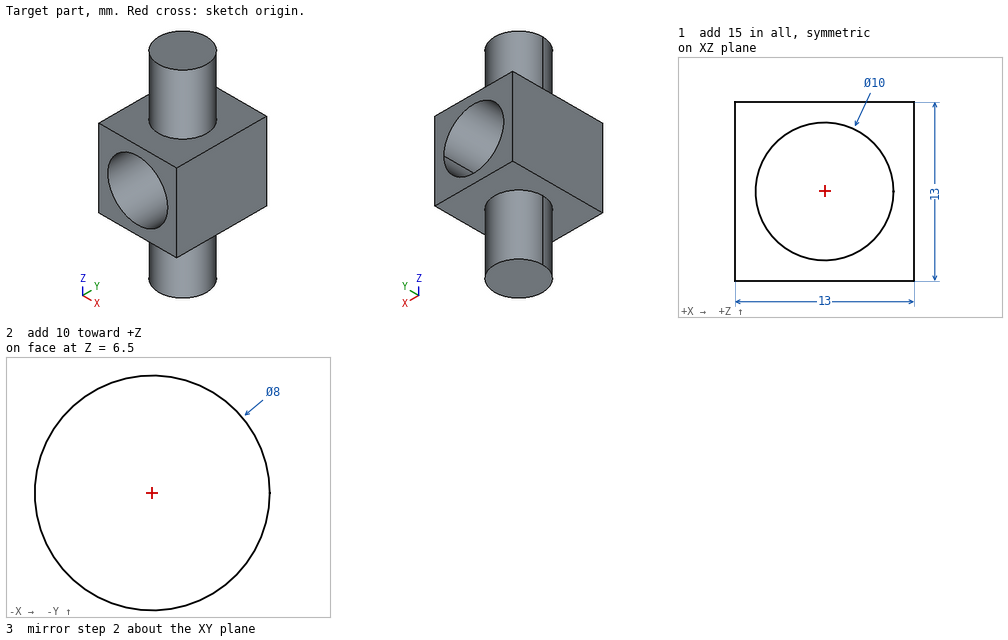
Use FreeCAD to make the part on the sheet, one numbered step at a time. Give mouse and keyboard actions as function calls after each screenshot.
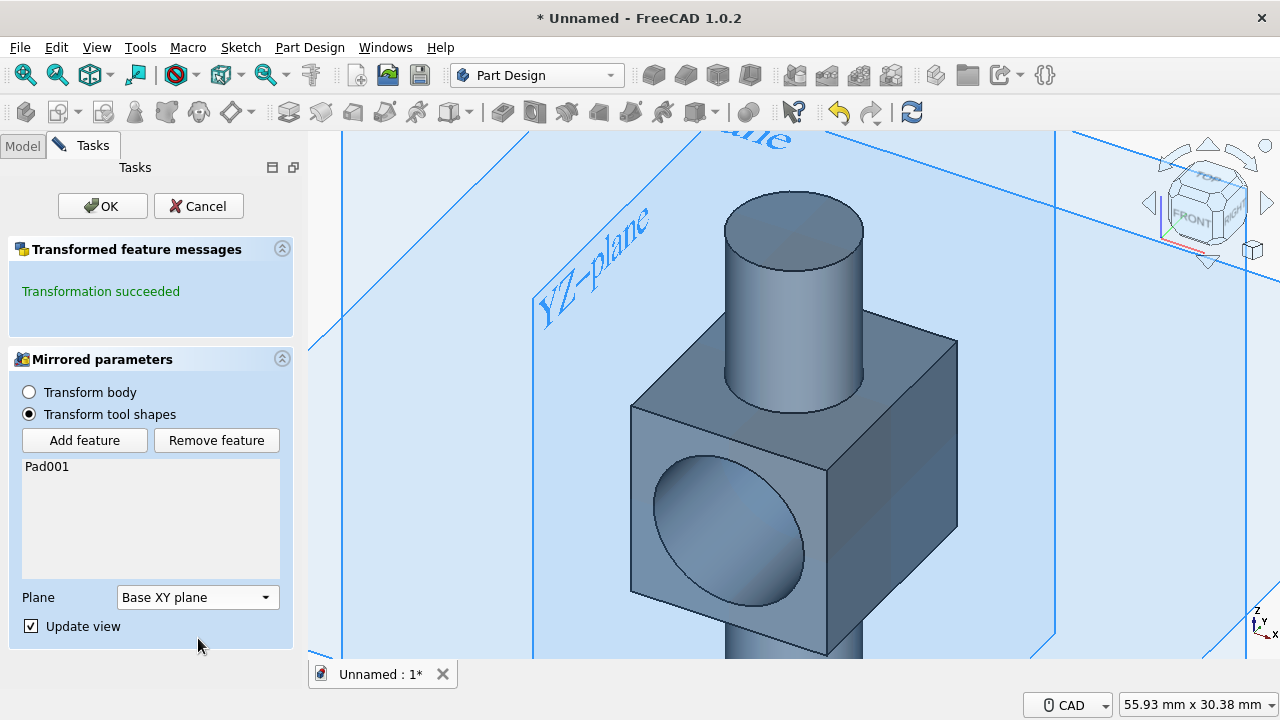
click(103, 206)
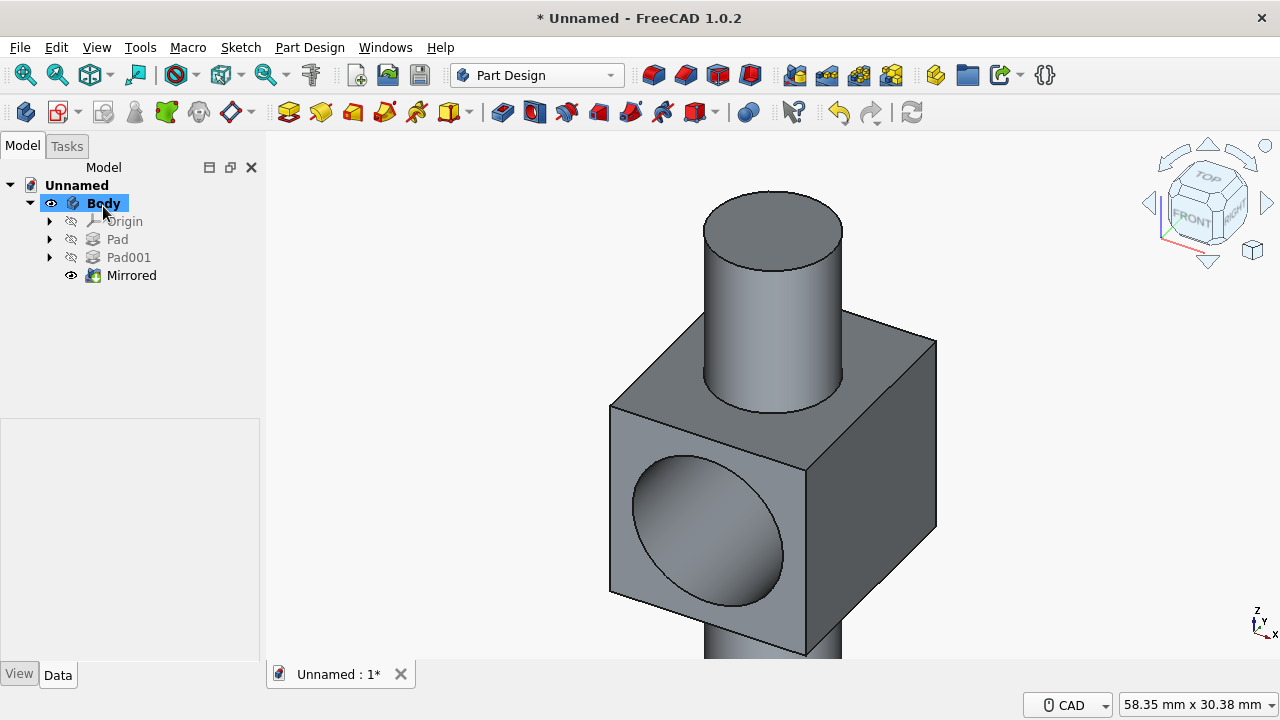
key(0)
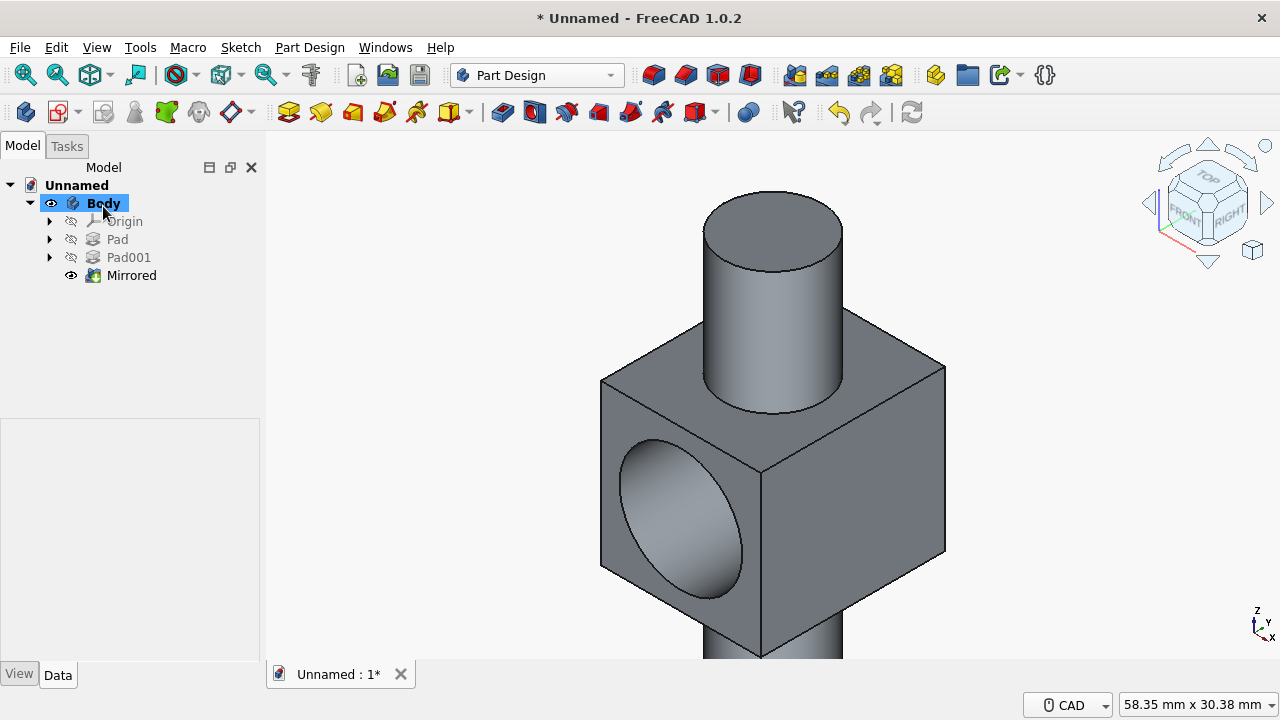
click(26, 76)